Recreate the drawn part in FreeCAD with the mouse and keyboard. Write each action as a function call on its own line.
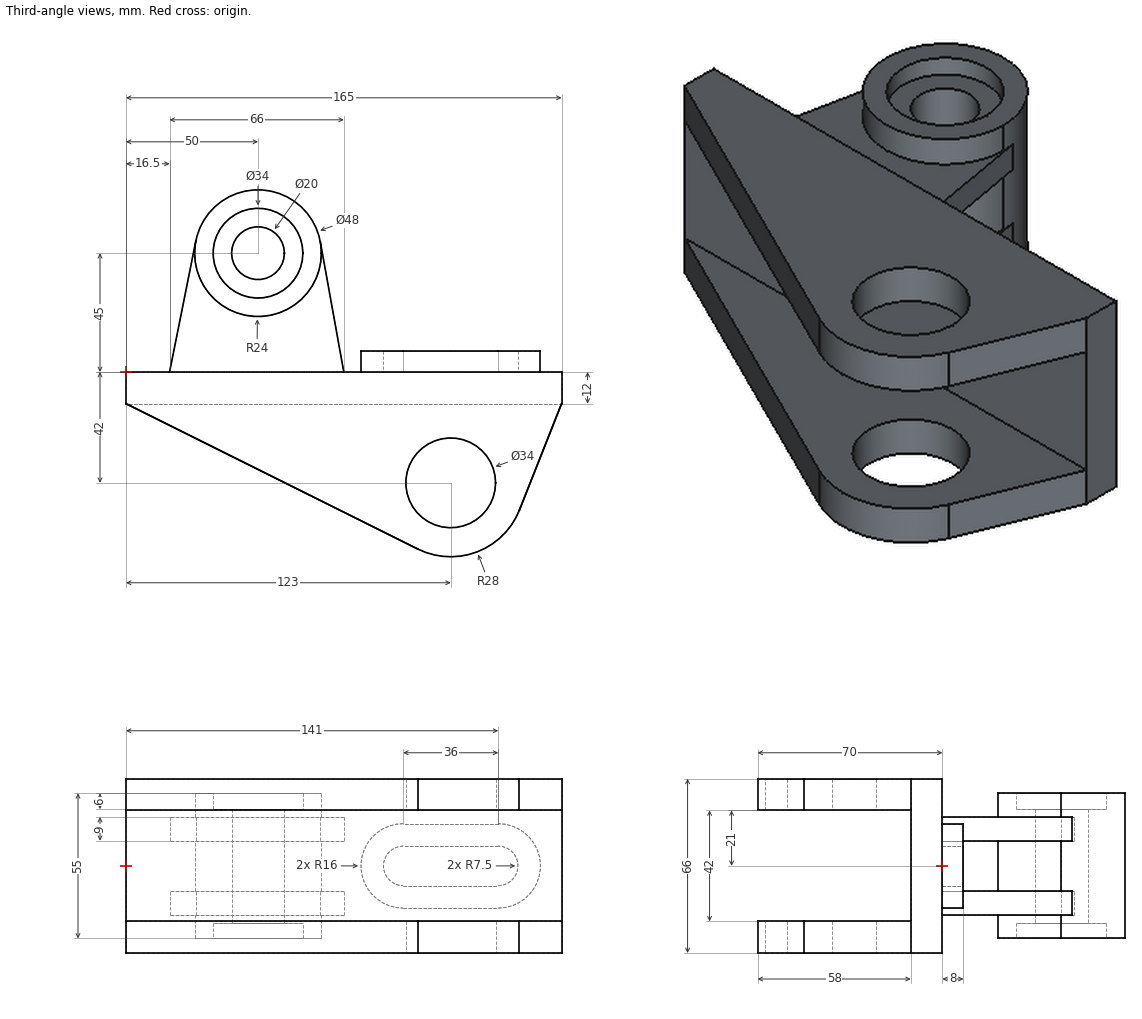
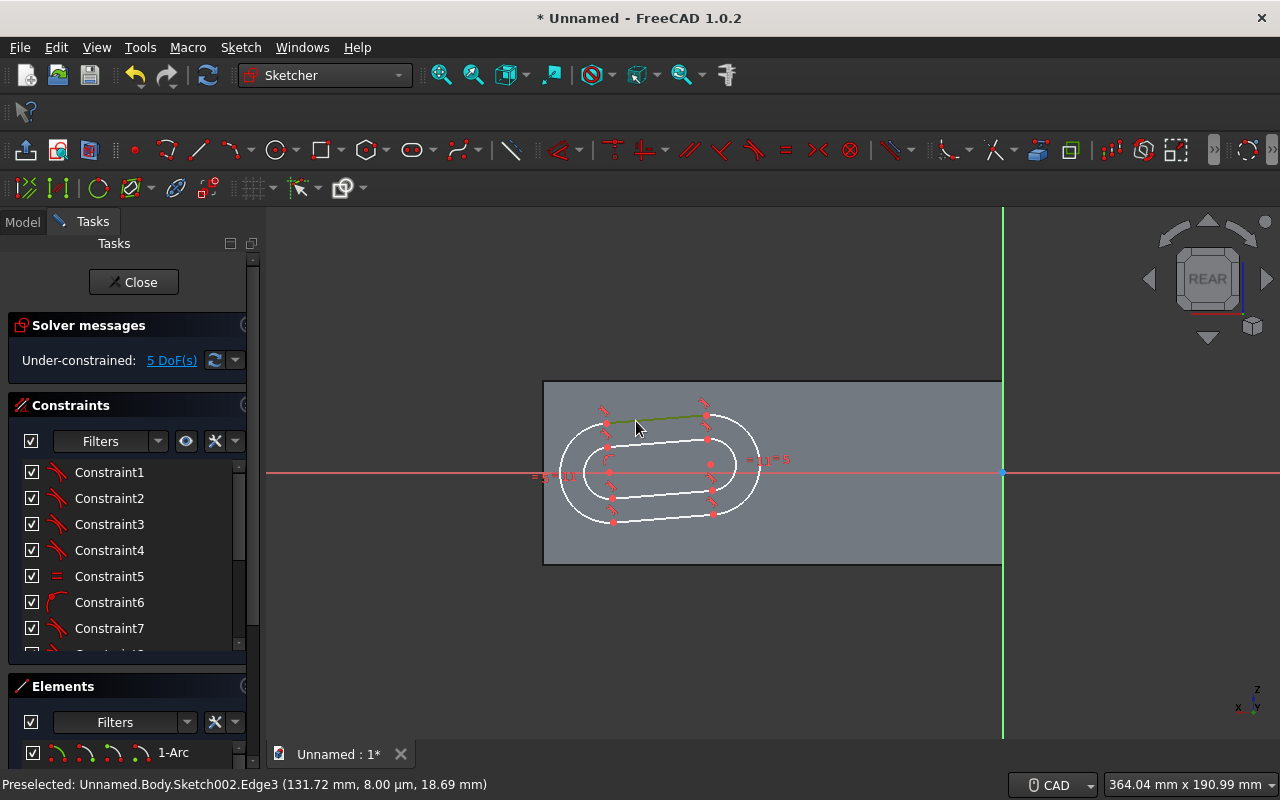
key(h)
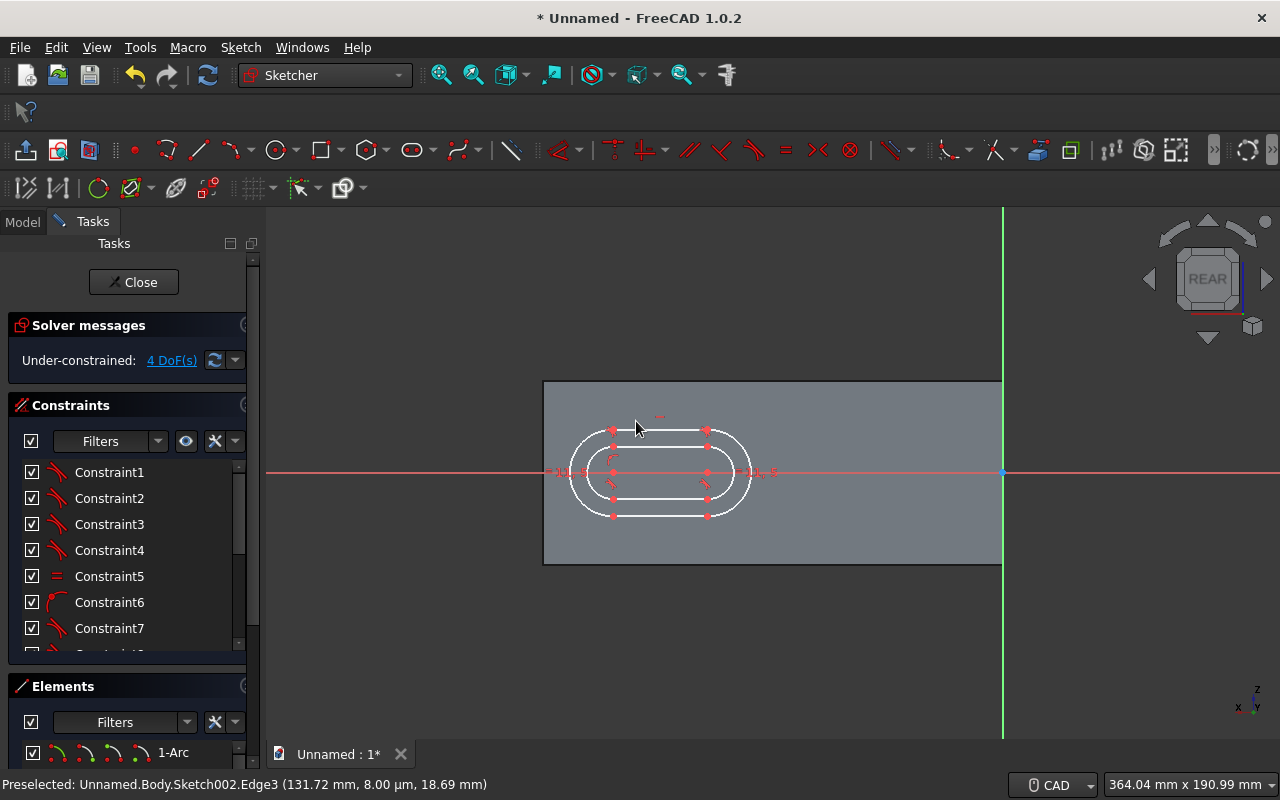
click(558, 150)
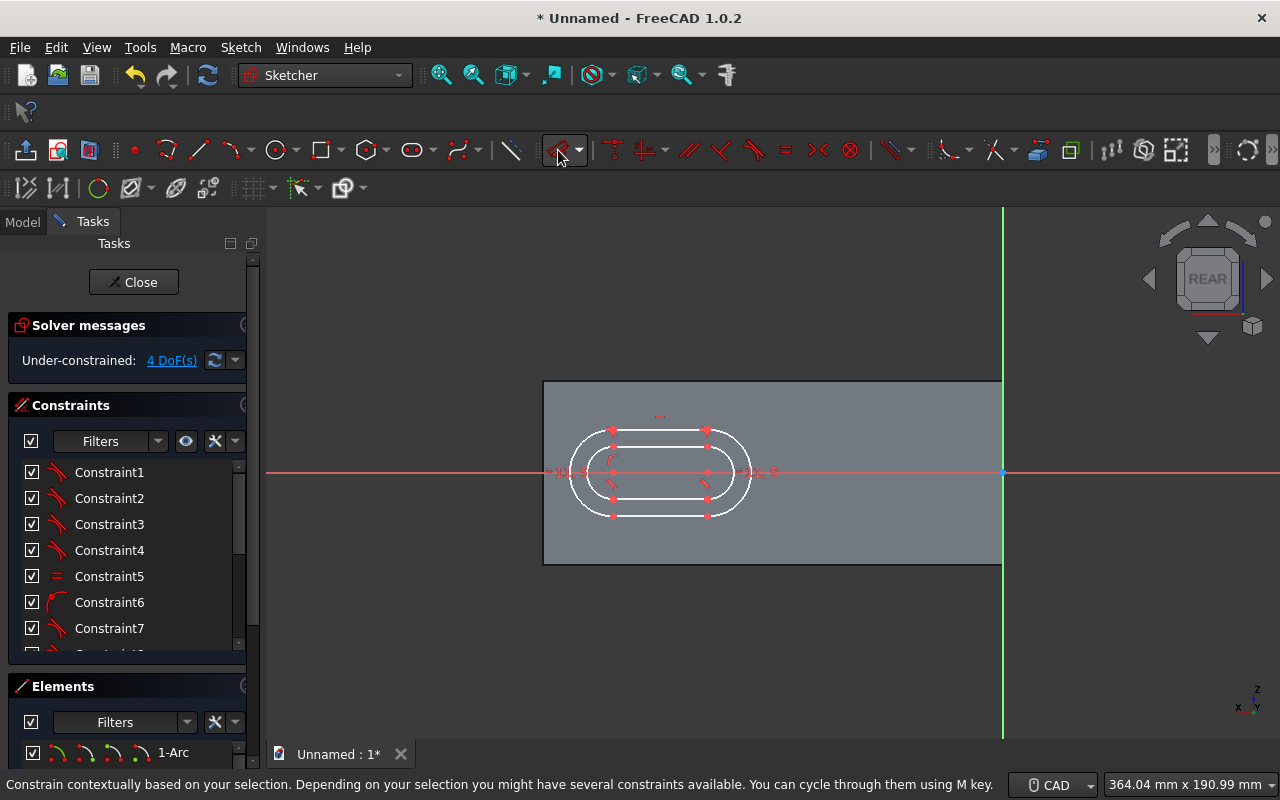
click(578, 448)
click(552, 429)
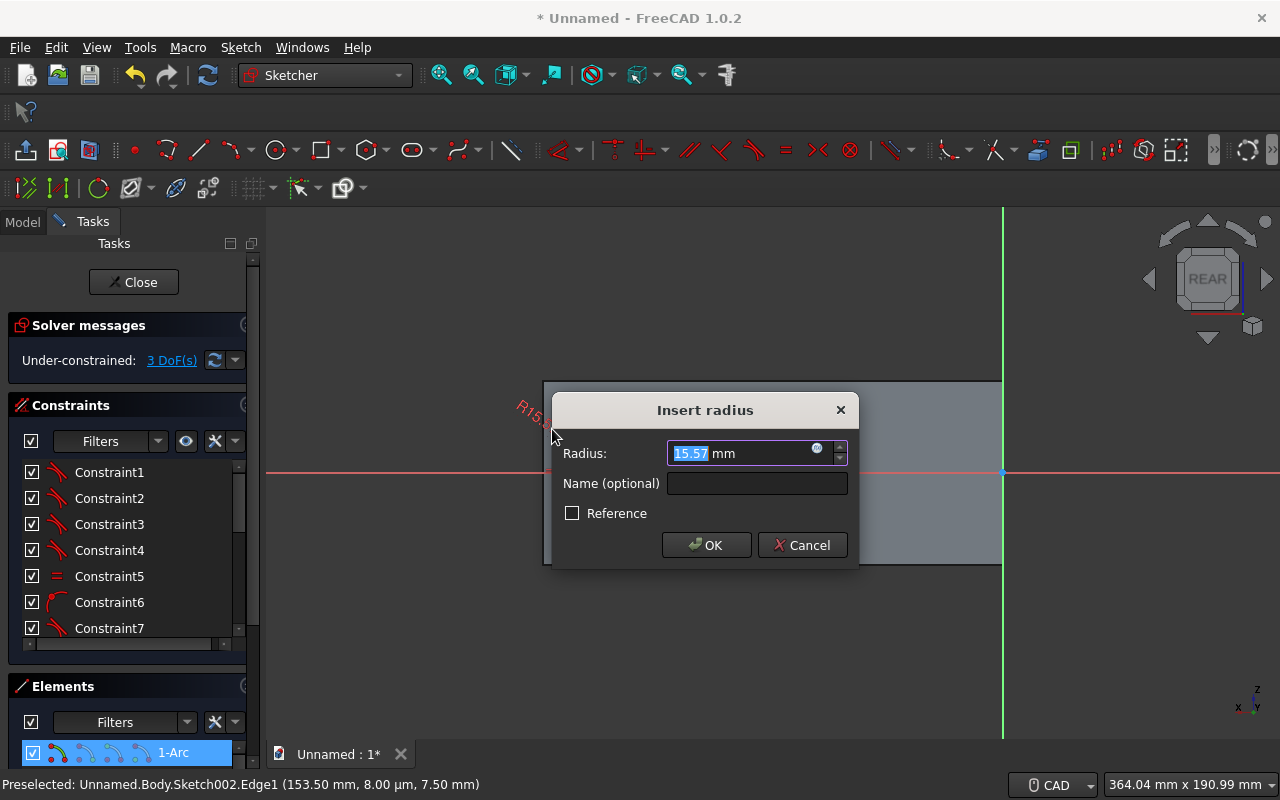
text(16)
key(Return)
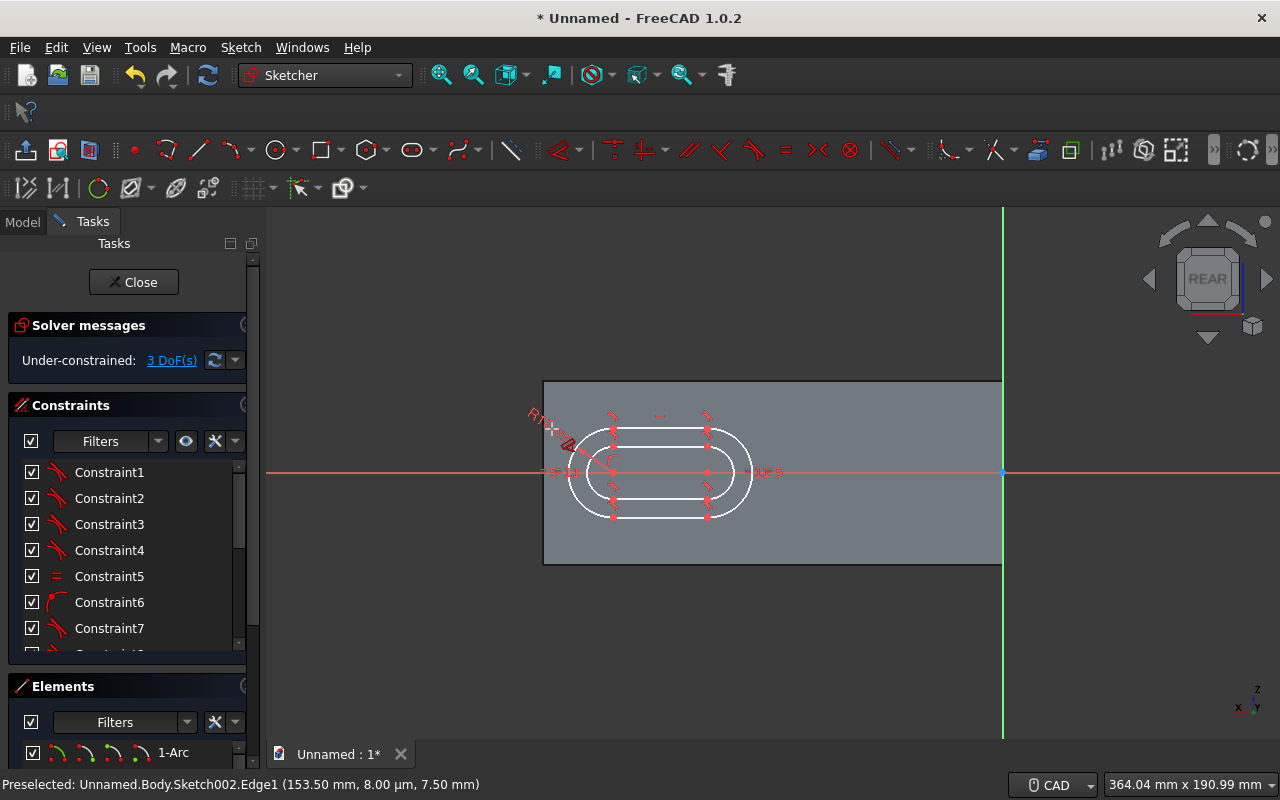
scroll(592, 458, up, 4)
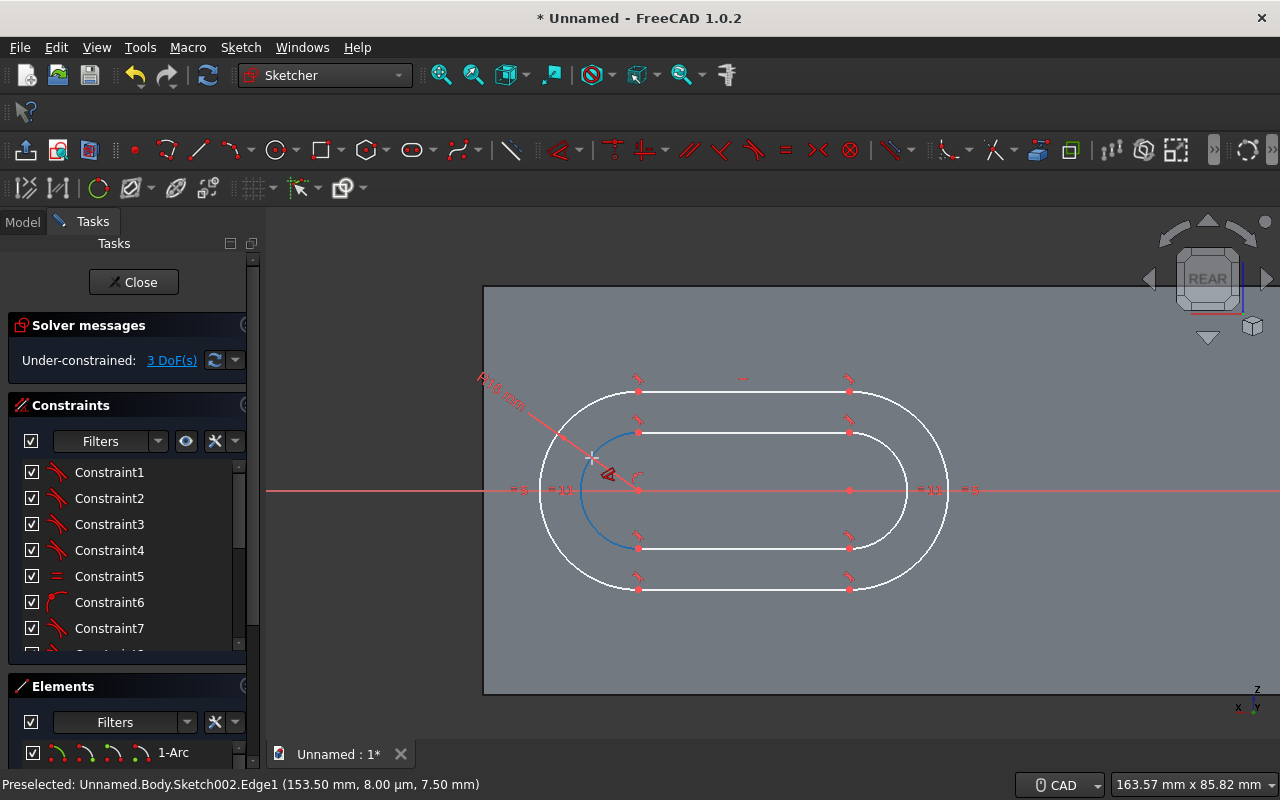
click(592, 457)
click(691, 418)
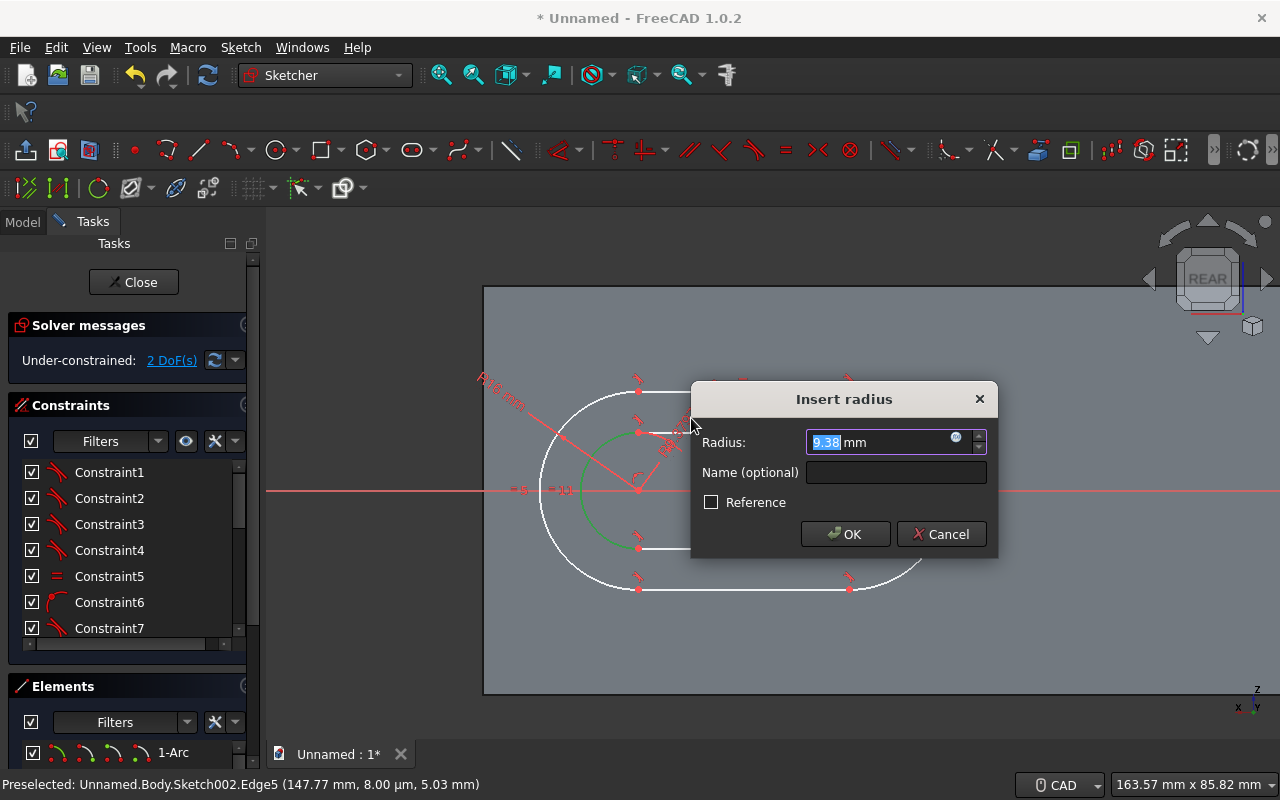
text(7.5)
key(Return)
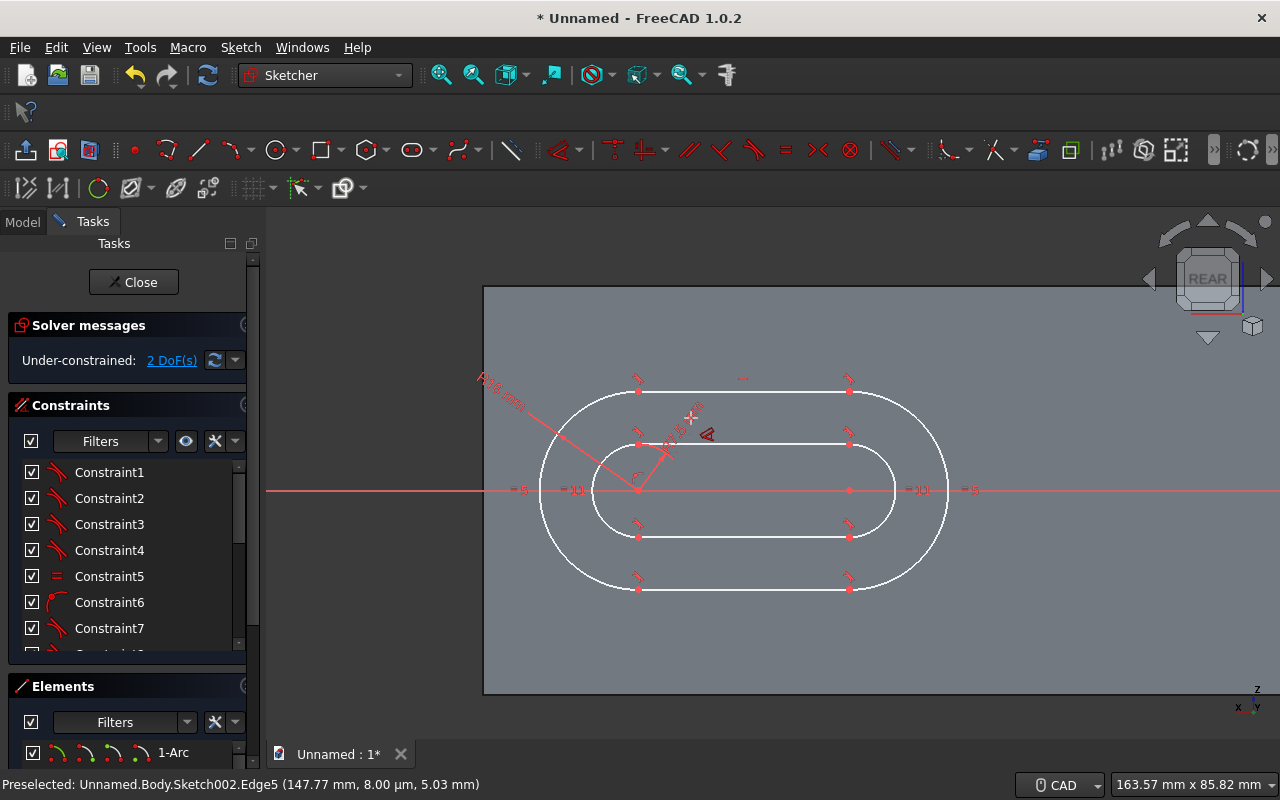
click(702, 392)
click(744, 358)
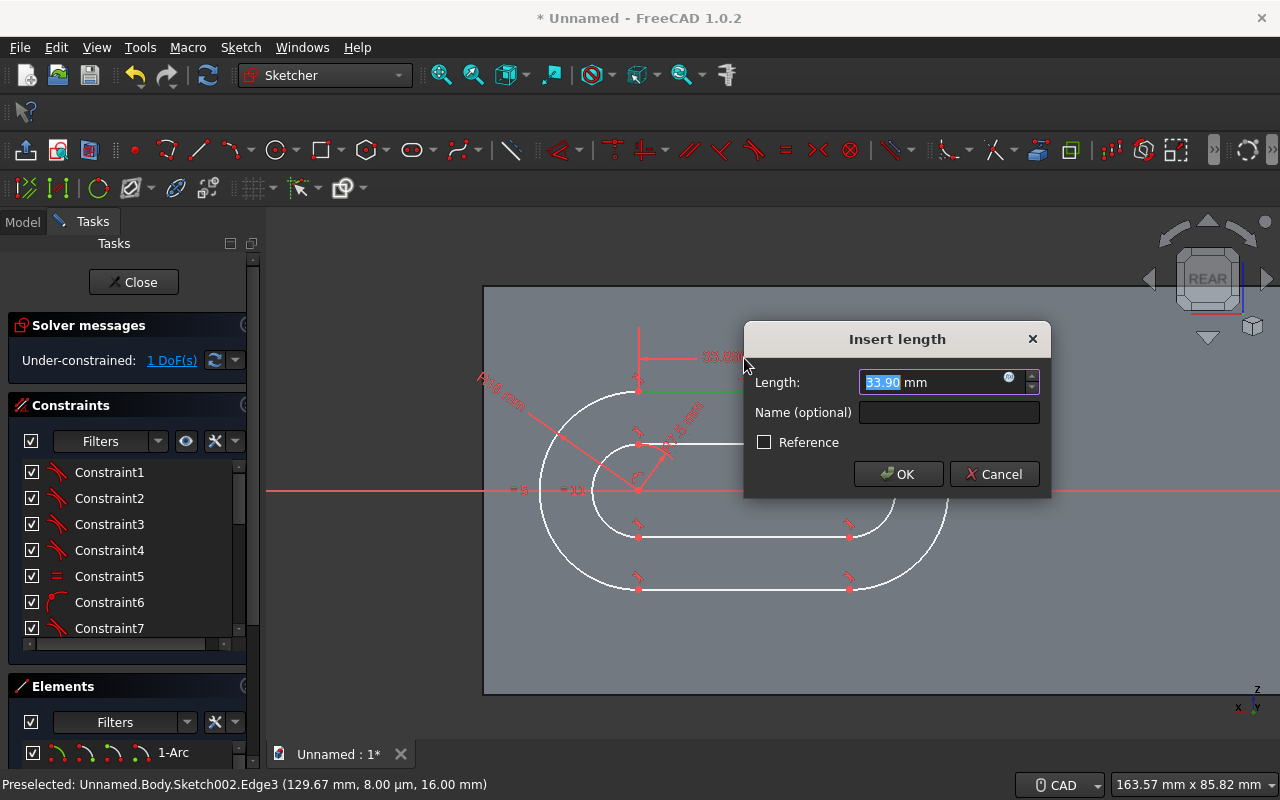
text(36)
key(Return)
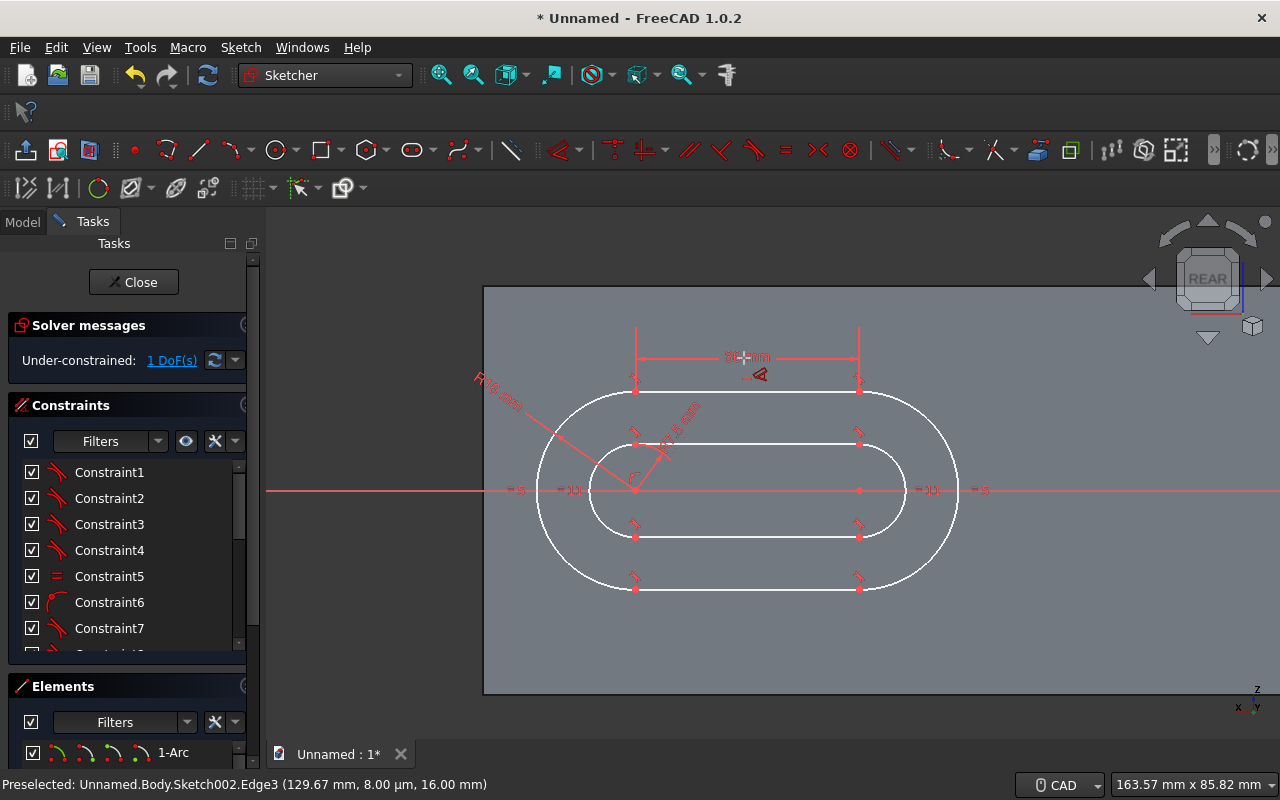
click(636, 392)
click(875, 358)